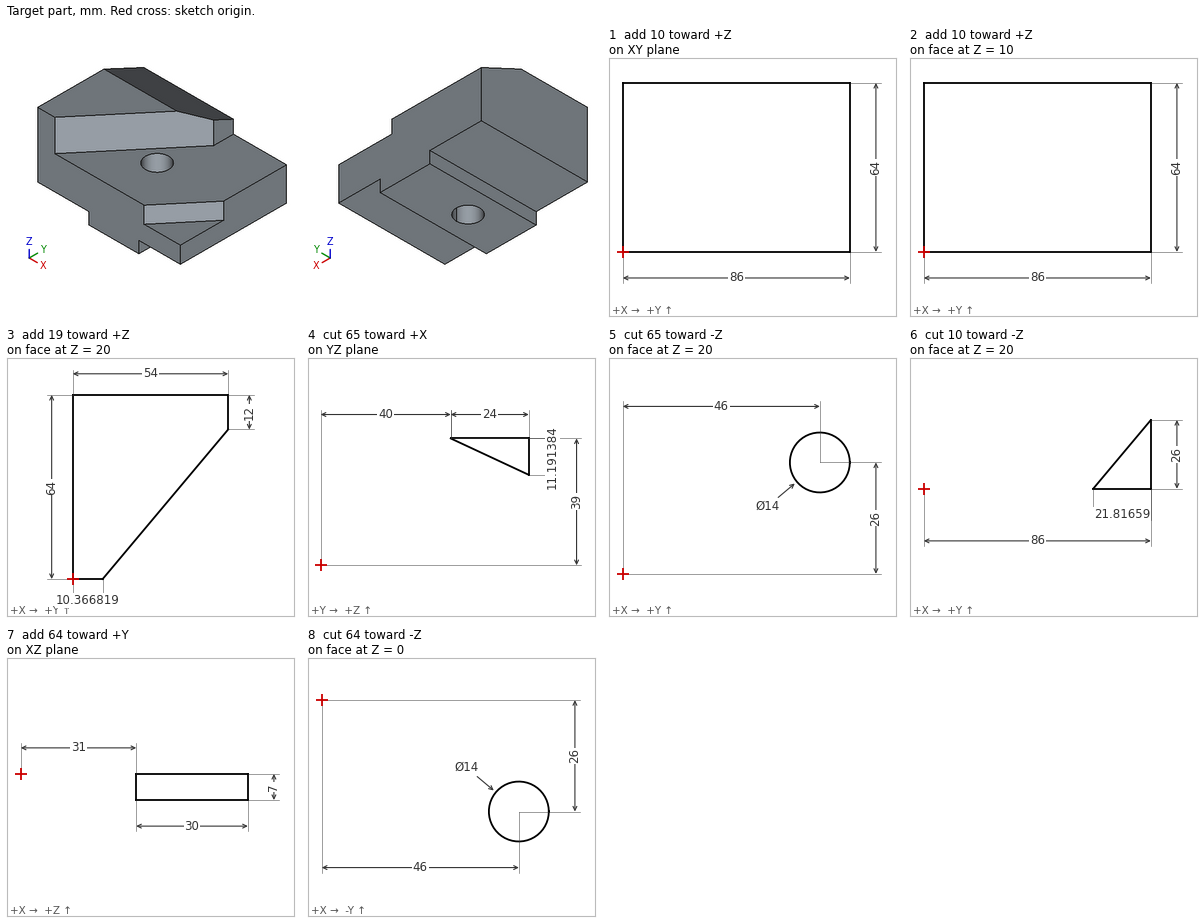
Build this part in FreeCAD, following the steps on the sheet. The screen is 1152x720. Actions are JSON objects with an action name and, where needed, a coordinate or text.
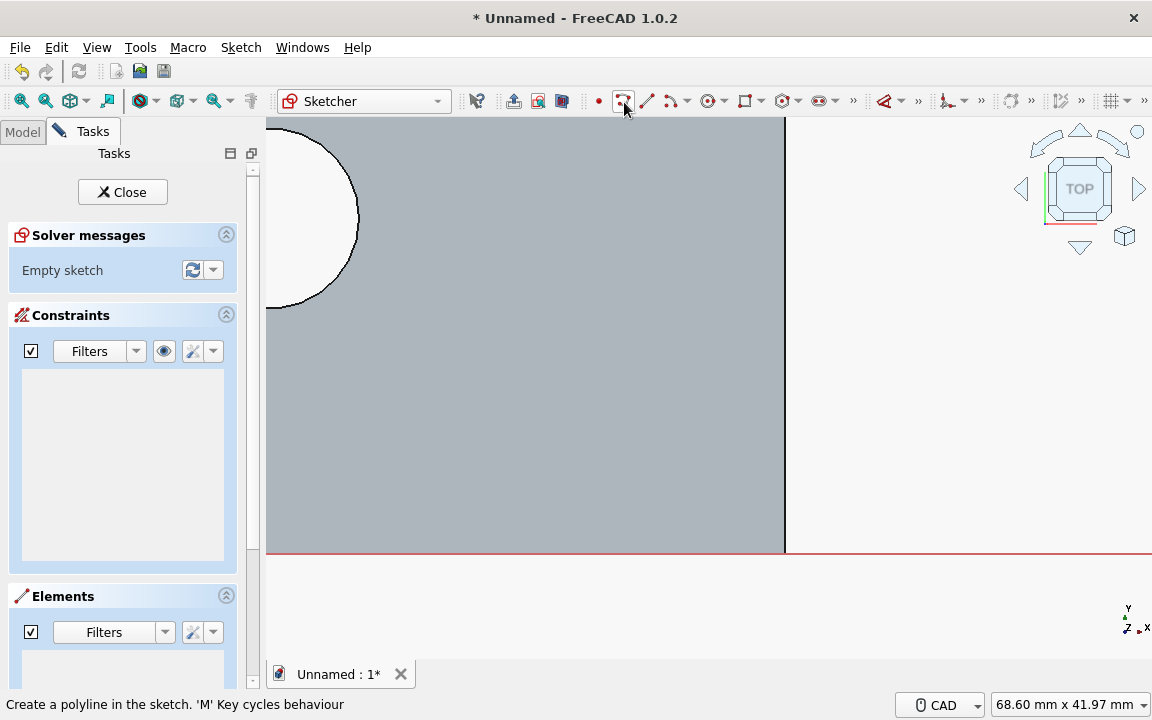
{"action": "left_click", "coordinate": [504, 554]}
{"action": "left_click", "coordinate": [785, 545]}
{"action": "left_click", "coordinate": [785, 218]}
{"action": "left_click", "coordinate": [504, 554]}
{"action": "key", "text": "Escape"}
{"action": "key", "text": "Escape"}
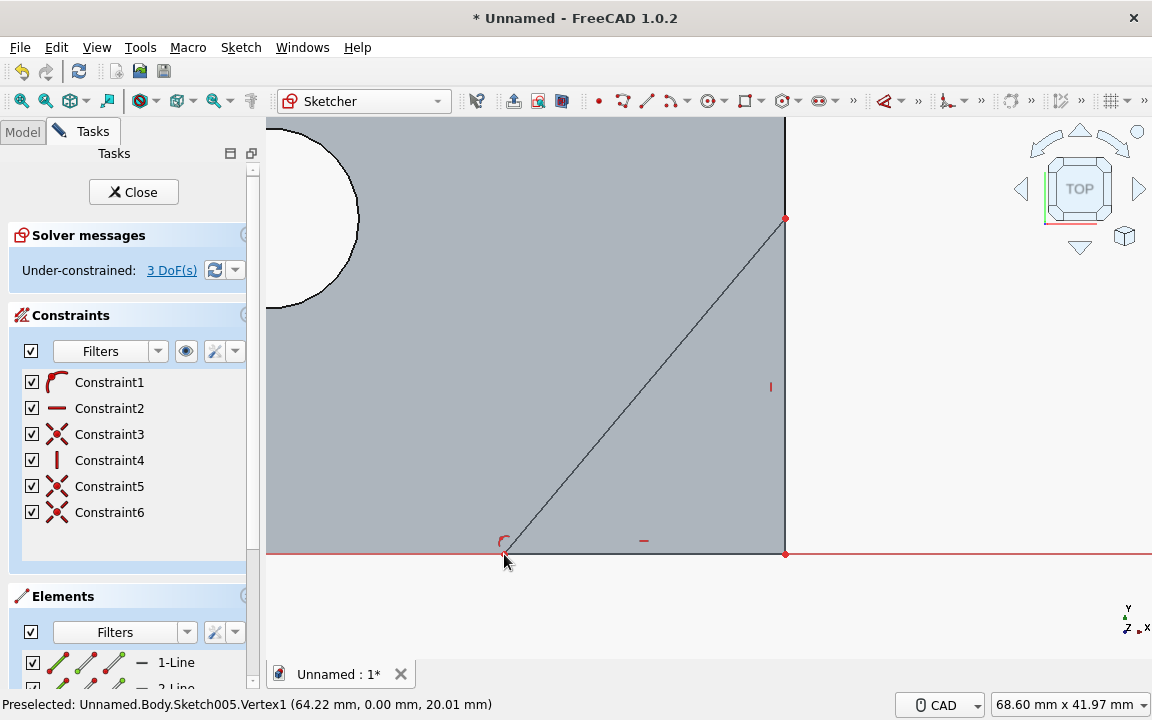
{"action": "left_click", "coordinate": [884, 102]}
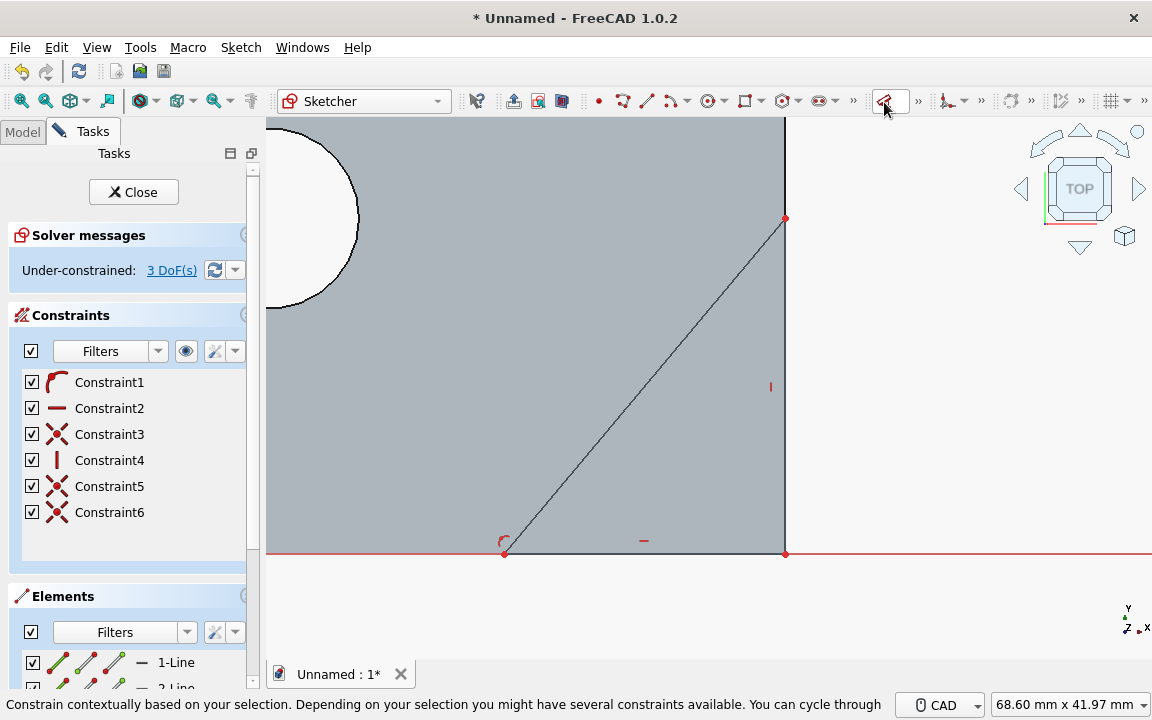
{"action": "left_click", "coordinate": [785, 454]}
{"action": "left_click", "coordinate": [819, 387]}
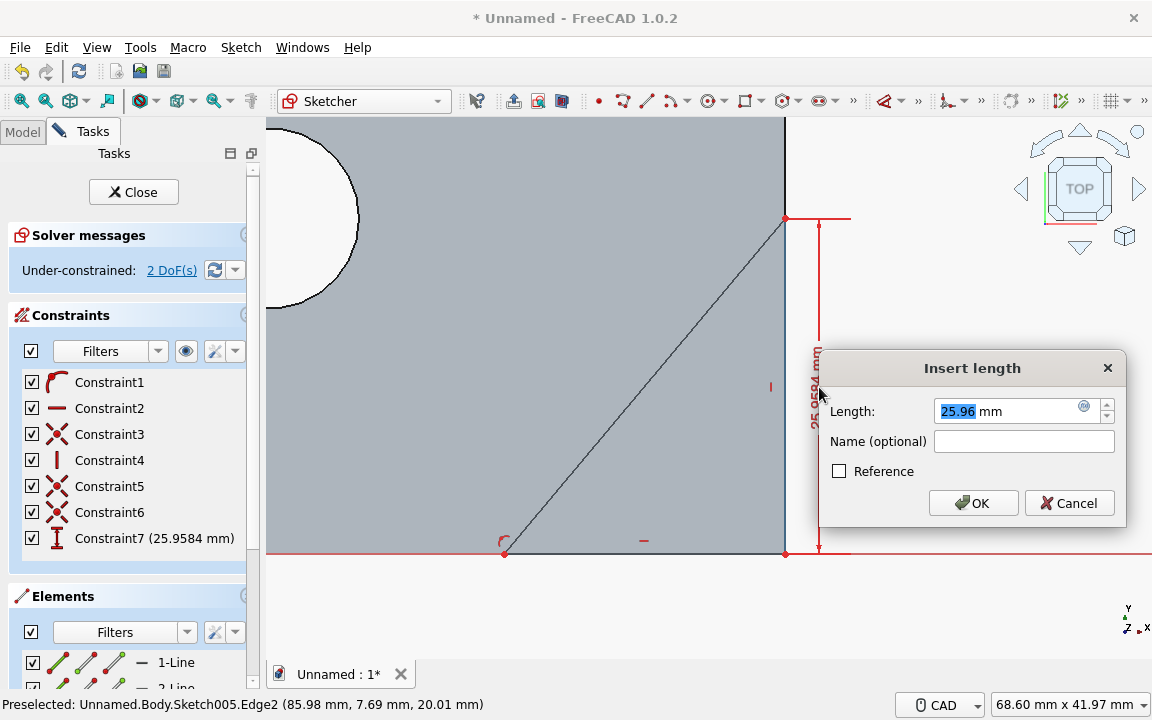
{"action": "type", "text": "26"}
{"action": "key", "text": "Return"}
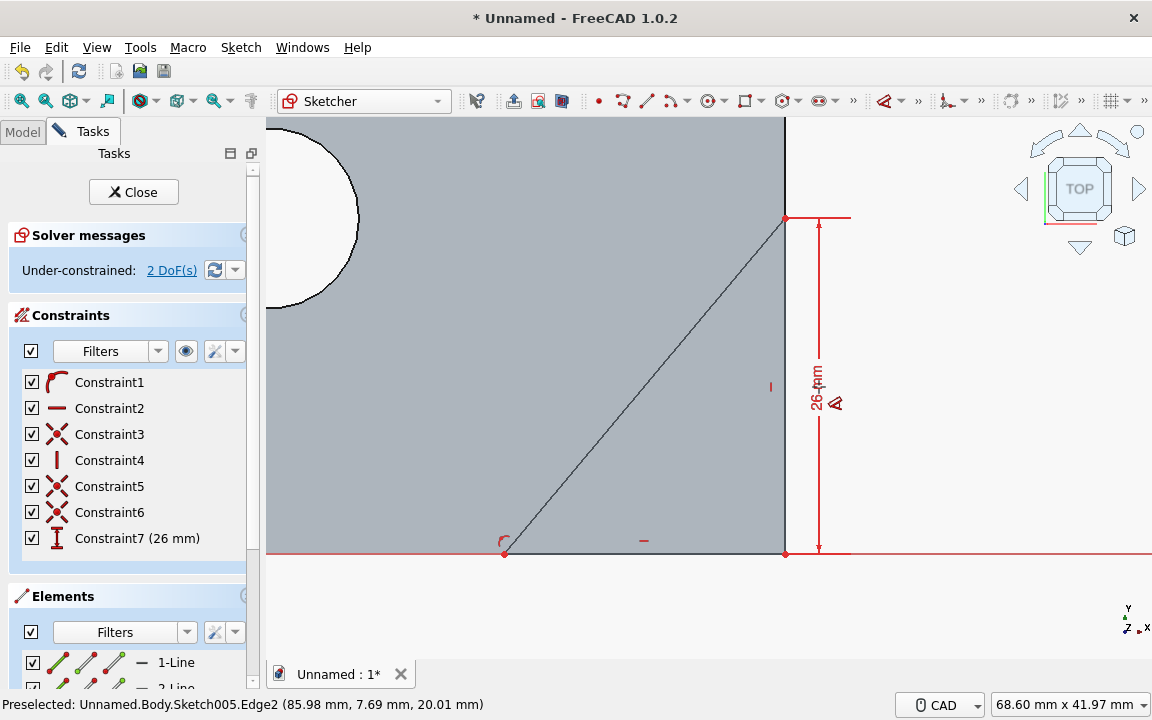
{"action": "left_click", "coordinate": [785, 554]}
{"action": "left_click", "coordinate": [539, 588]}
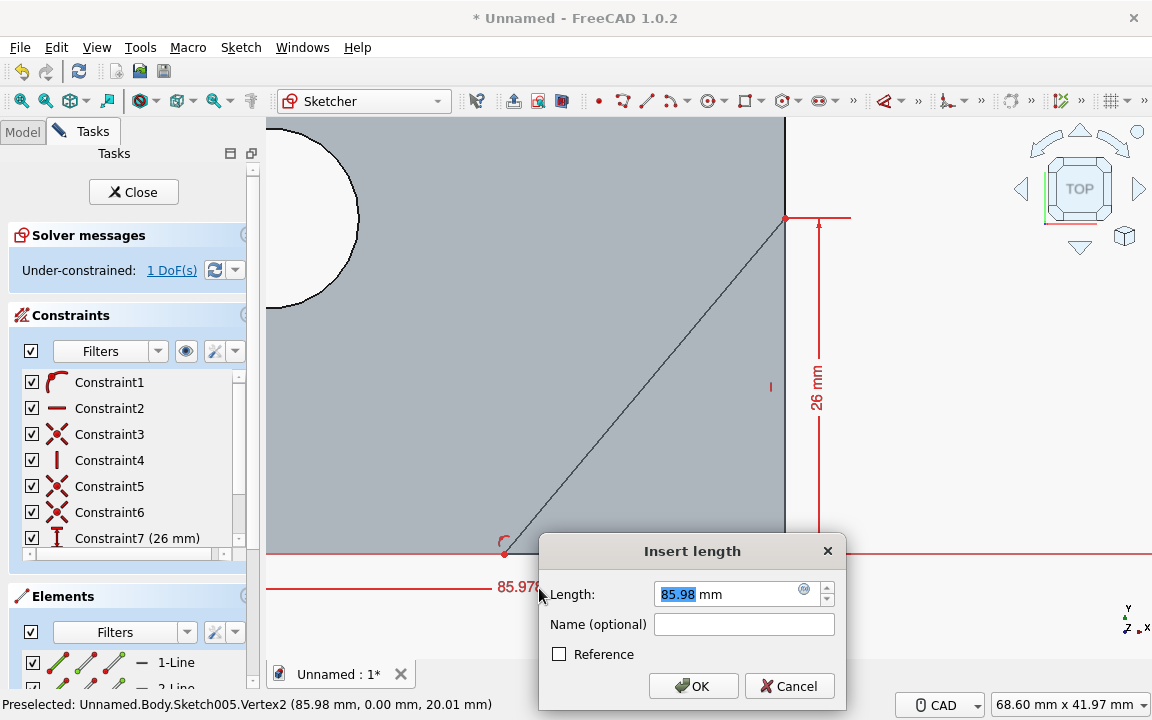
{"action": "type", "text": "86"}
{"action": "key", "text": "Return"}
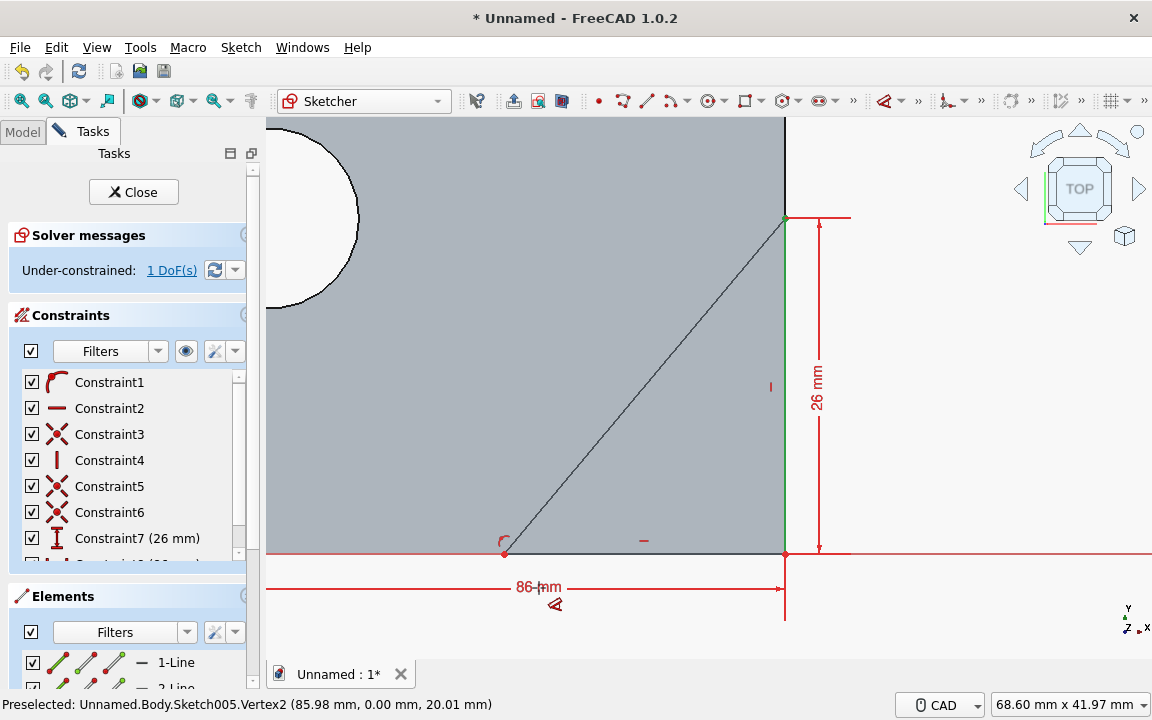
{"action": "left_click", "coordinate": [588, 554]}
{"action": "left_click", "coordinate": [645, 588]}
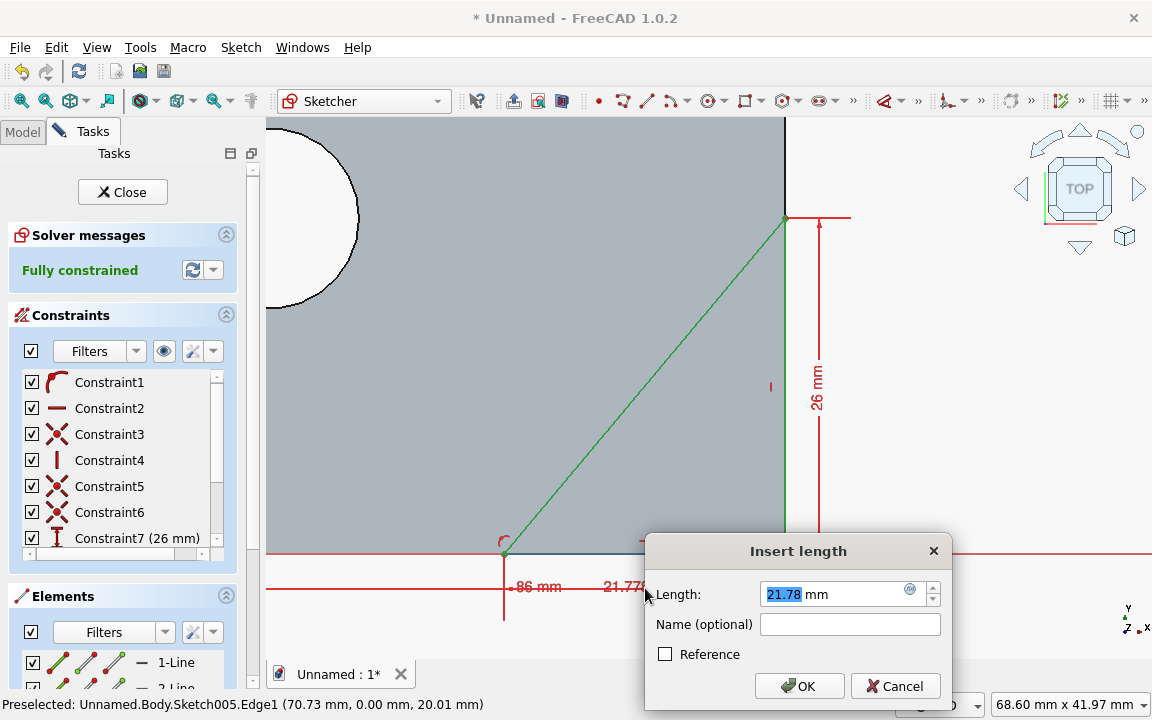
{"action": "type", "text": "21.81659"}
{"action": "key", "text": "Return"}
{"action": "key", "text": "Escape"}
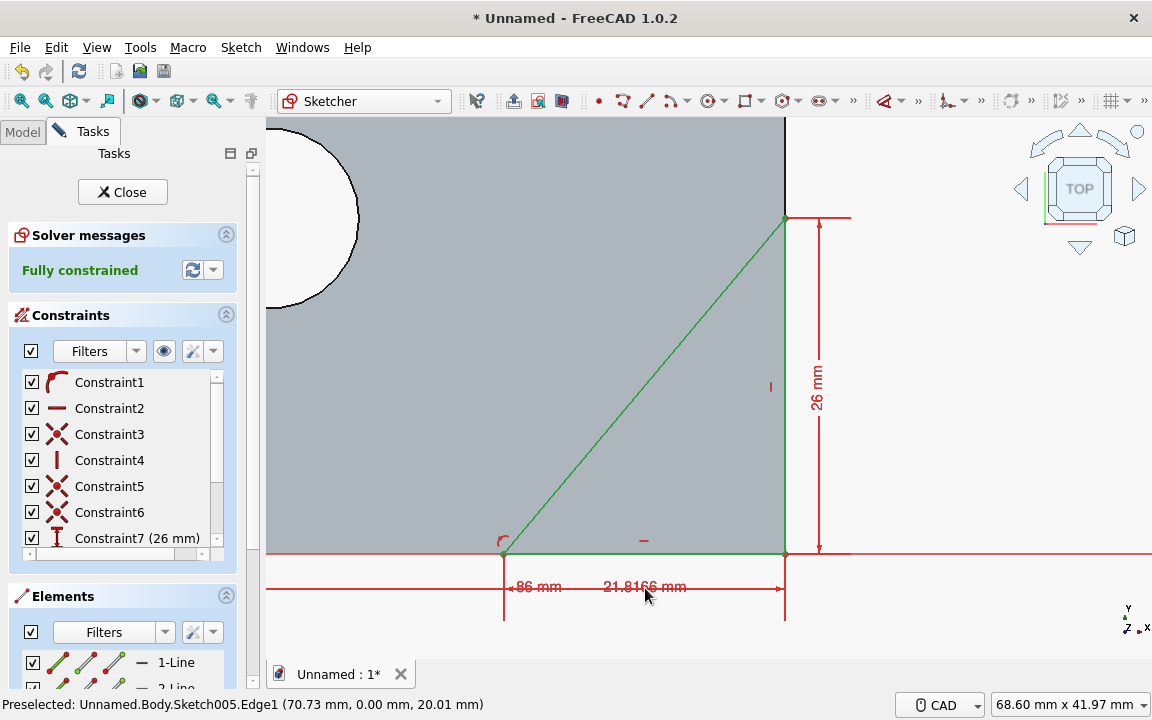
{"action": "left_click", "coordinate": [123, 192]}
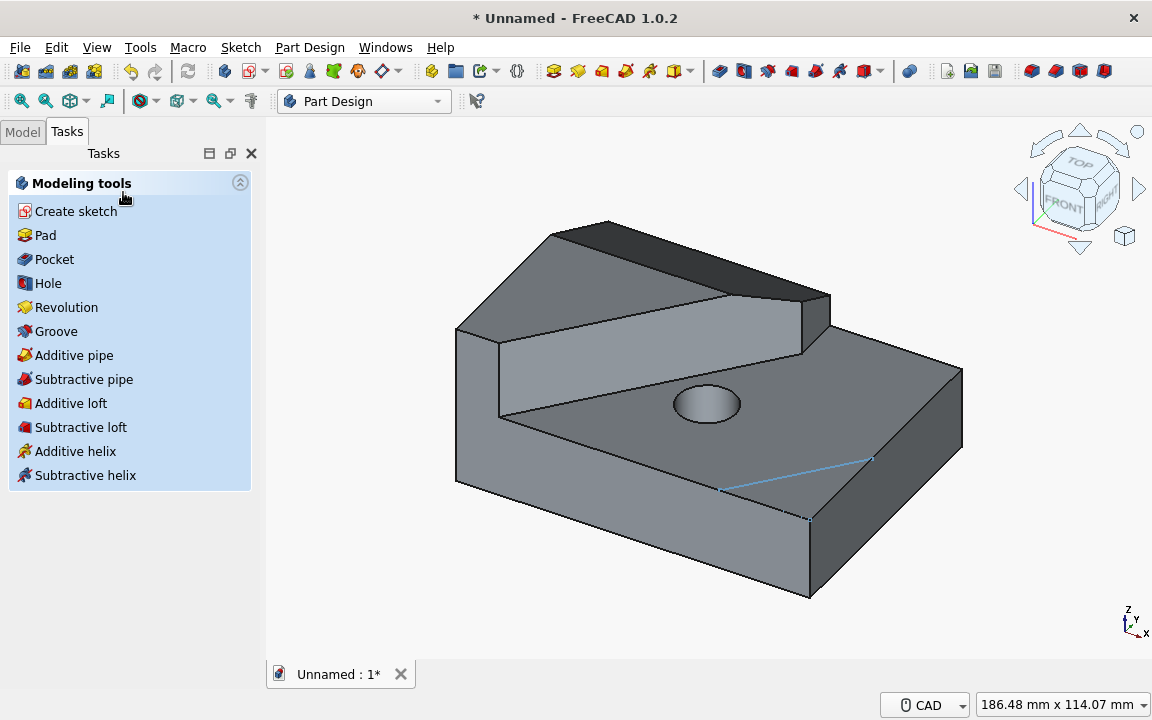
{"action": "left_click", "coordinate": [720, 72]}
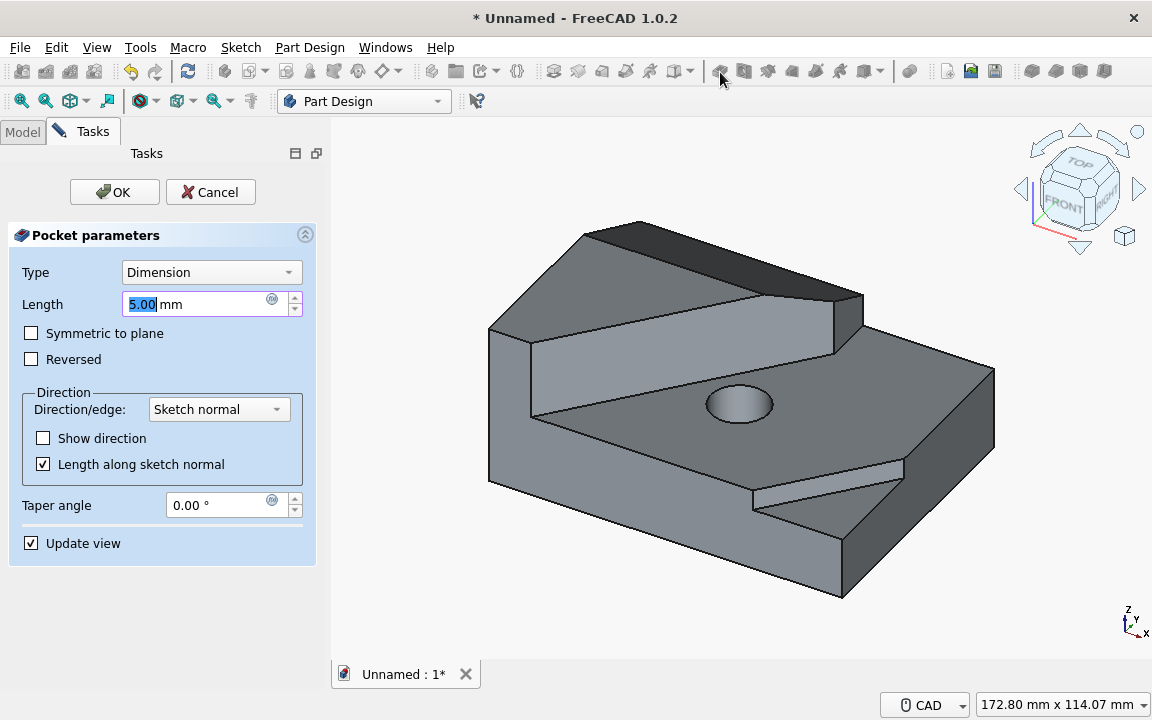
{"action": "type", "text": "10"}
{"action": "key", "text": "Tab"}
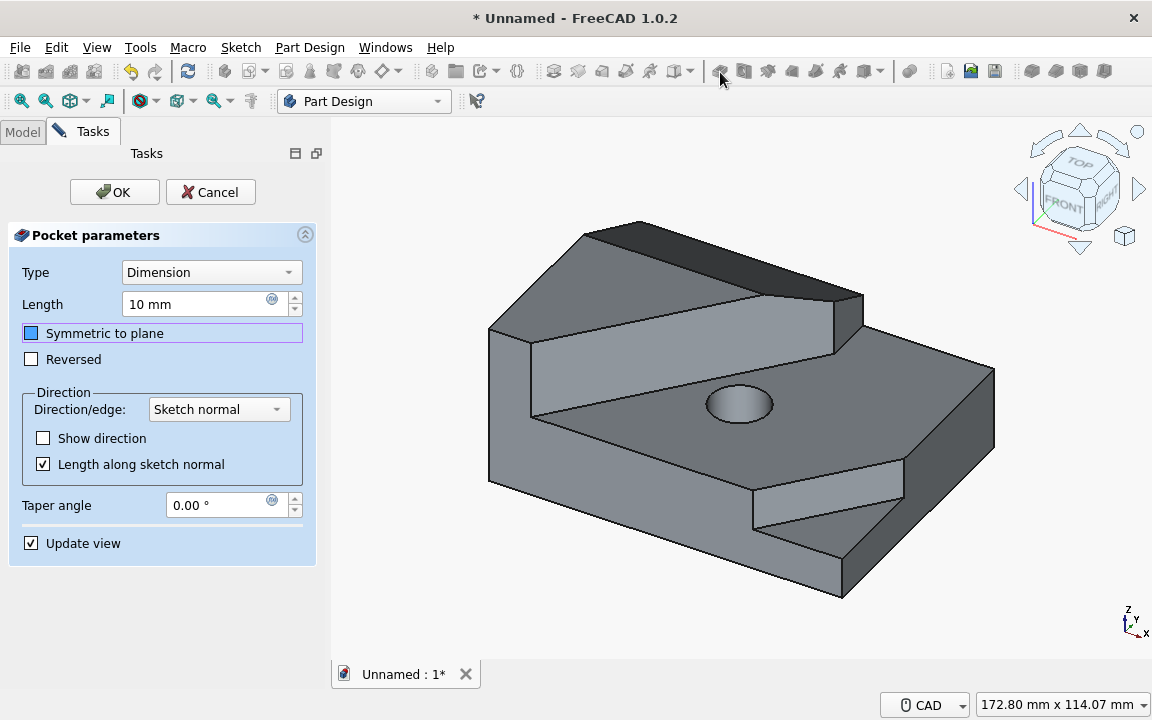
{"action": "left_click", "coordinate": [115, 192]}